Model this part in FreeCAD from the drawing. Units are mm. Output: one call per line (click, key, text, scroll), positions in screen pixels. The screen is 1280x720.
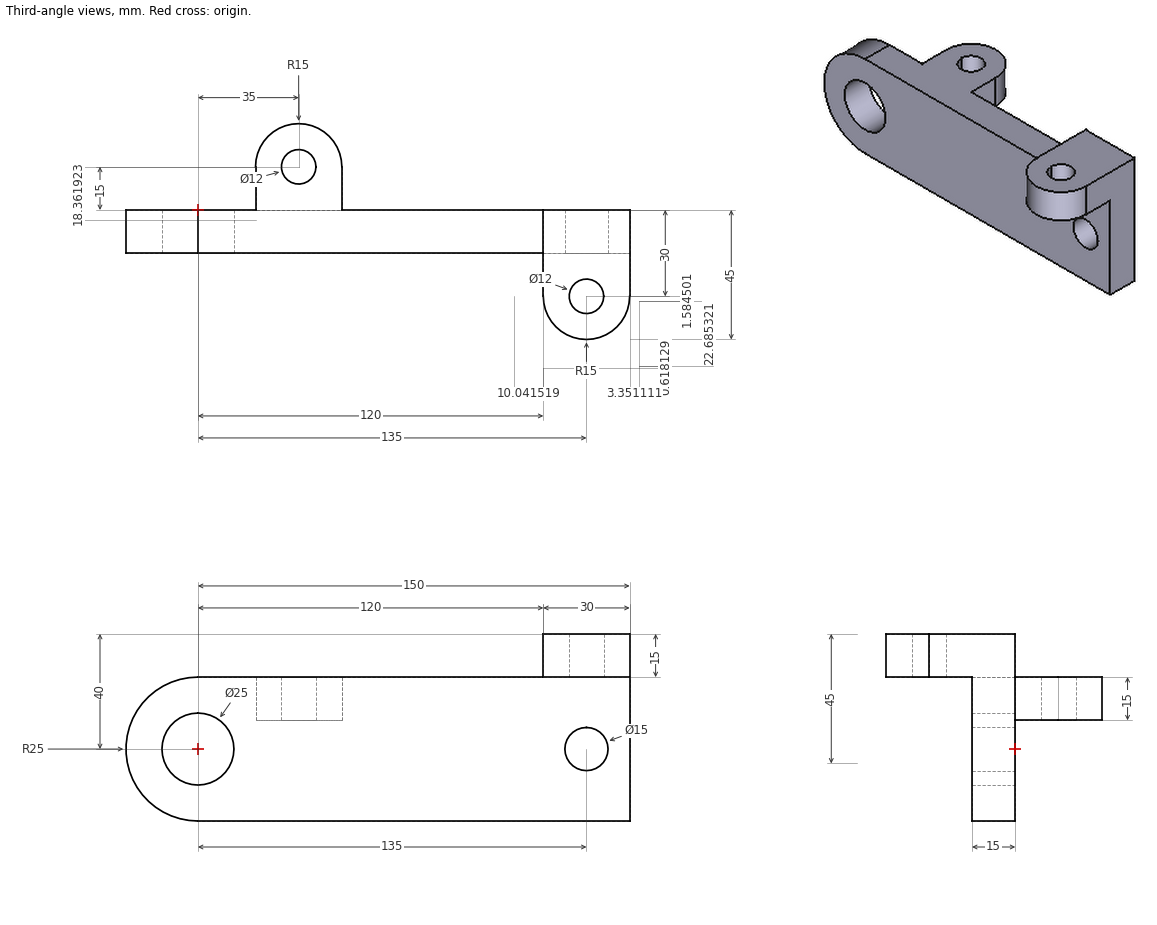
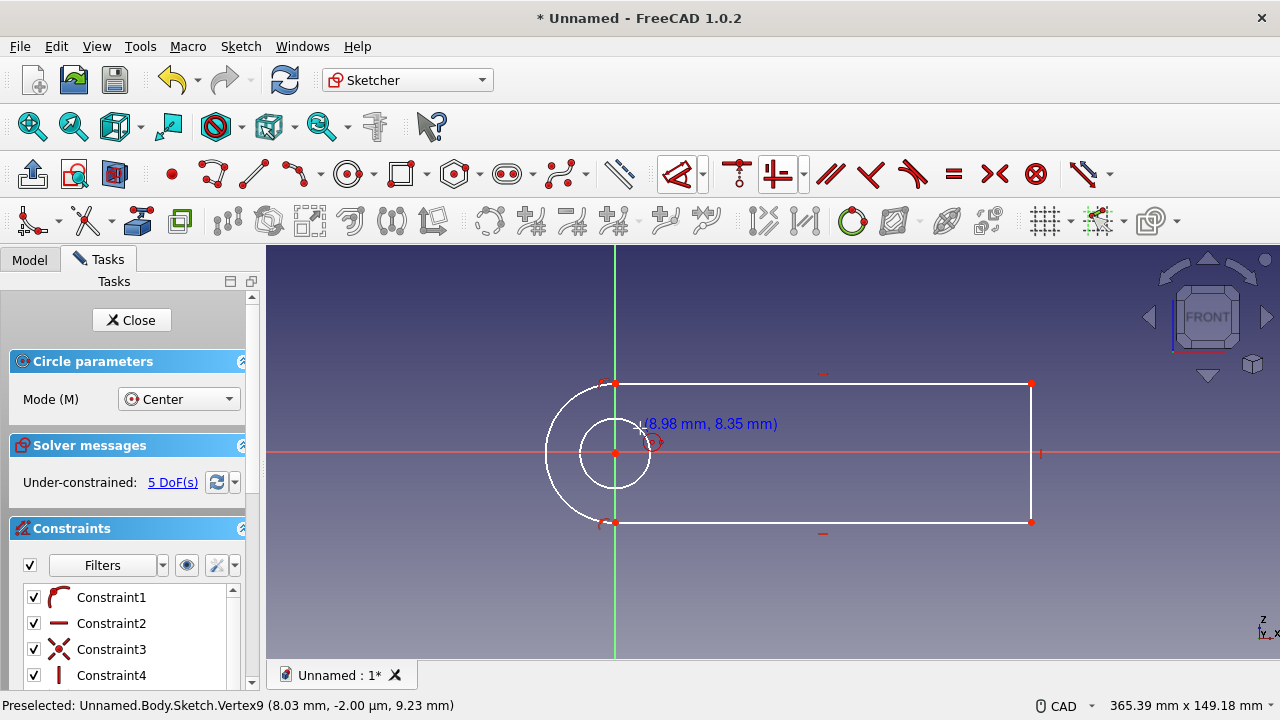
click(990, 452)
click(1004, 437)
key(Escape)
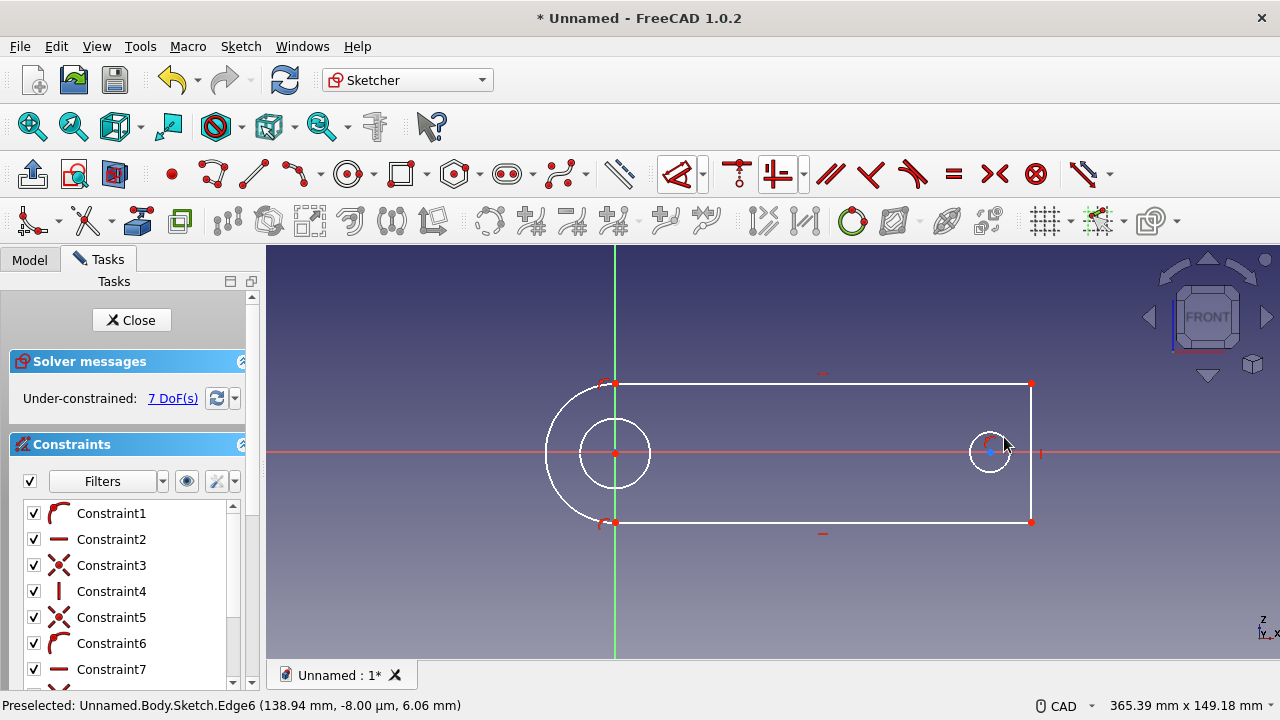
scroll(615, 453, up, 4)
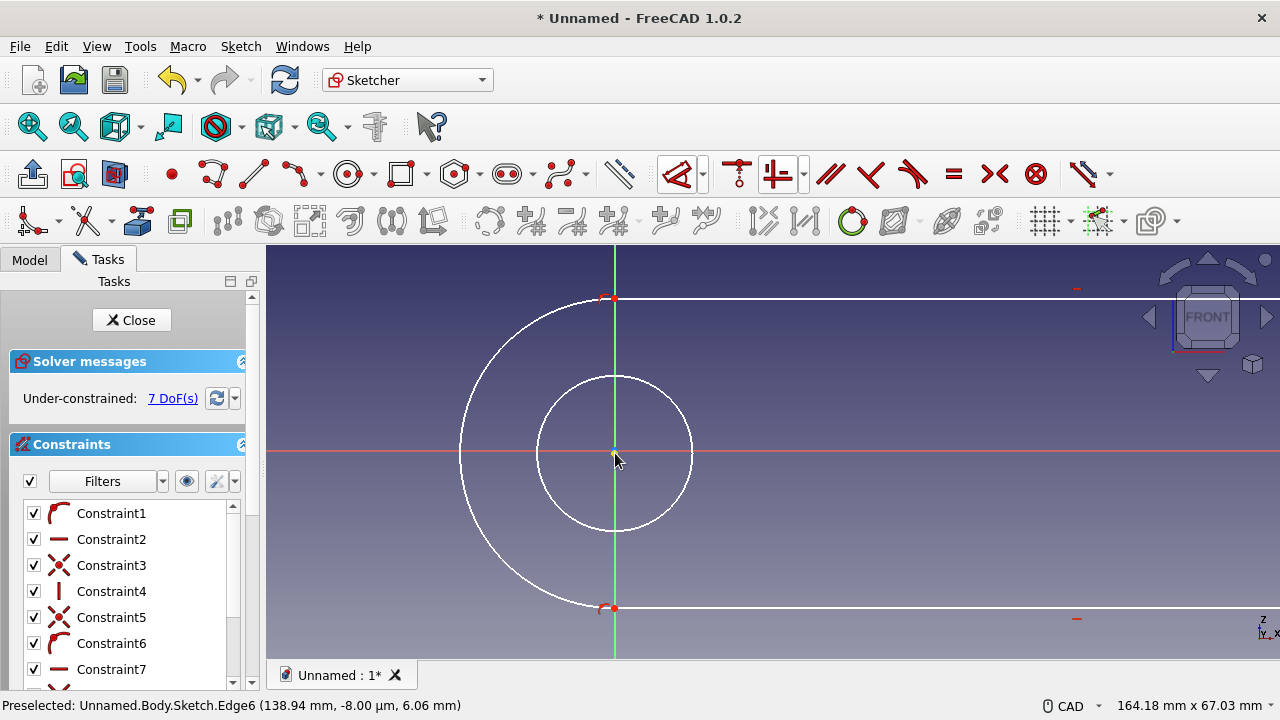
drag(605, 441, 625, 463)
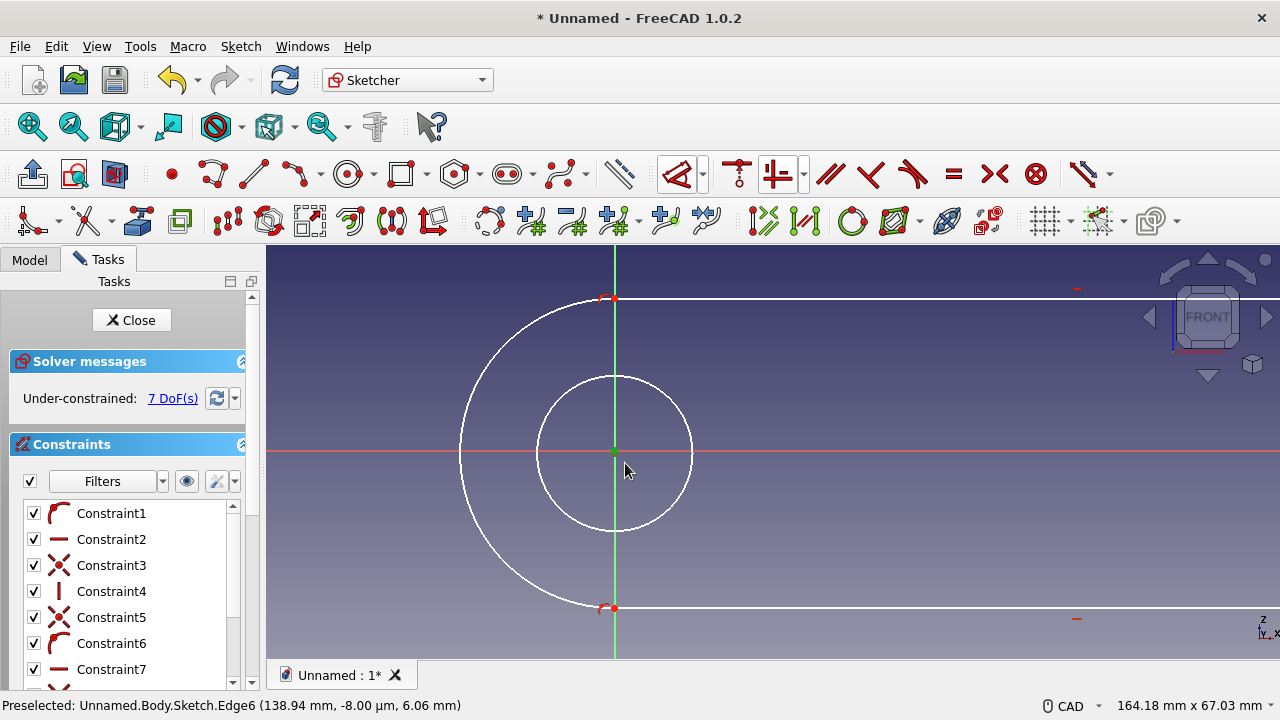
click(737, 174)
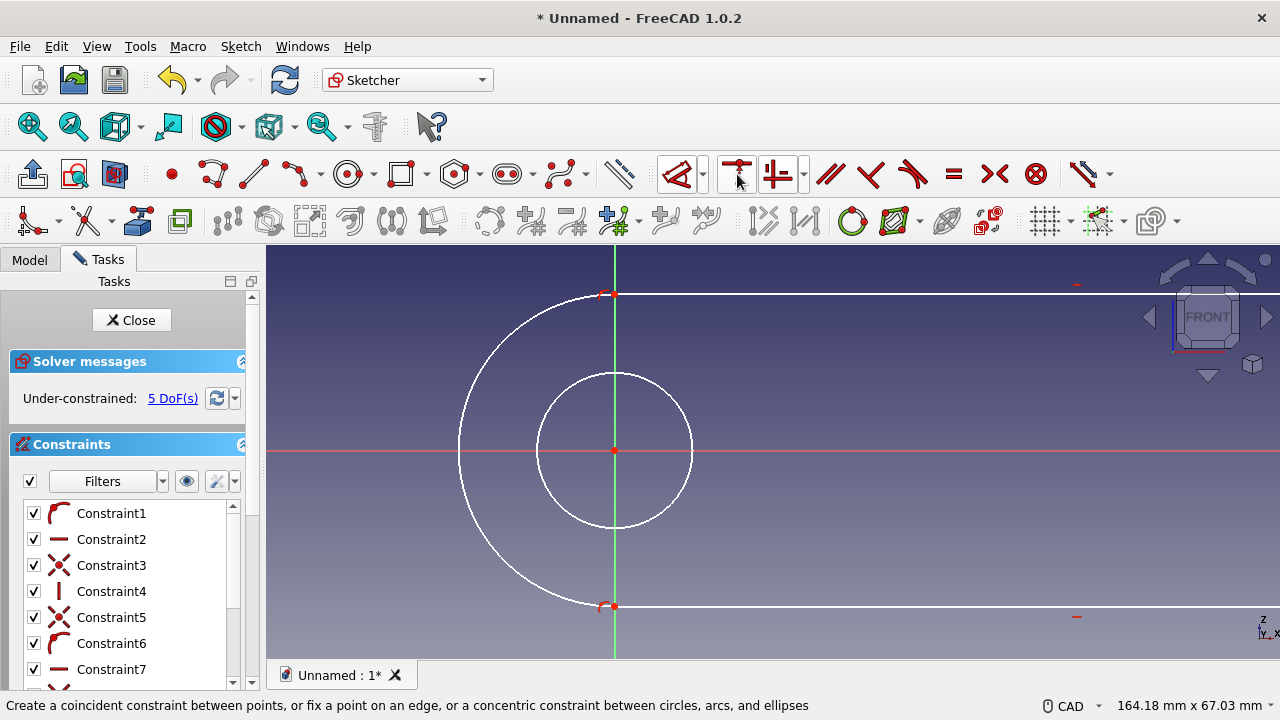
click(488, 359)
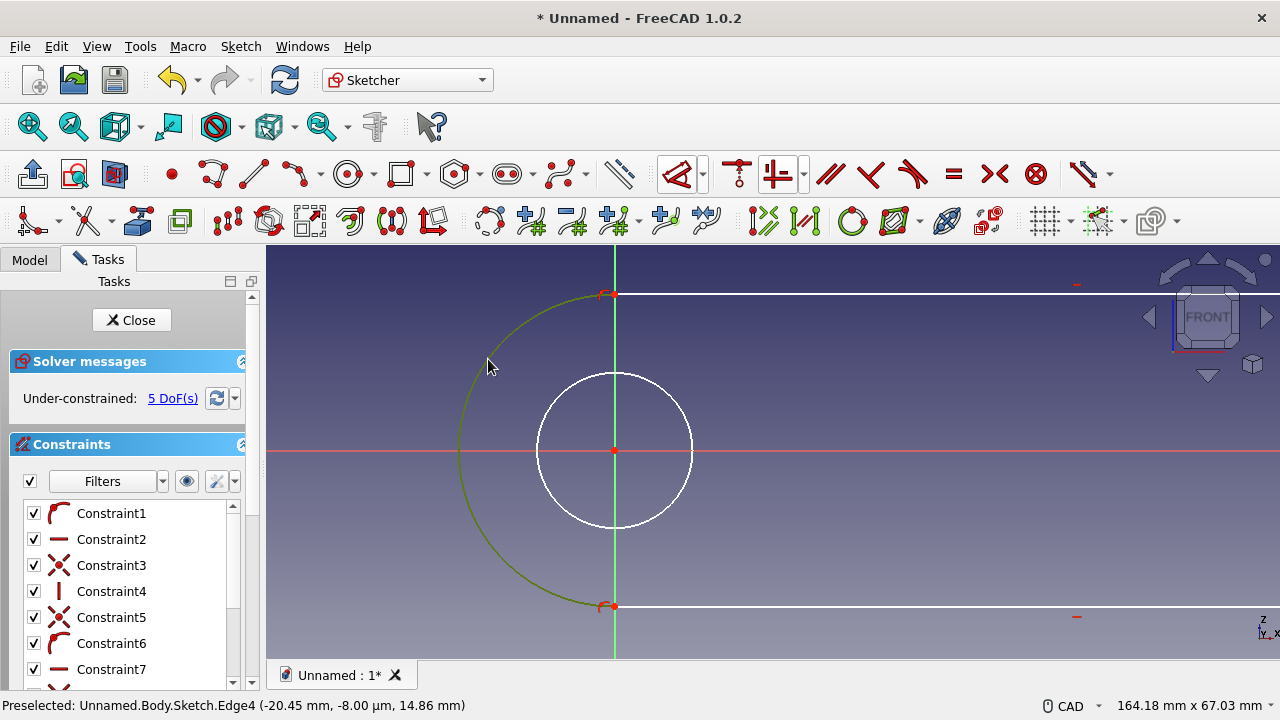
key(k)
key(r)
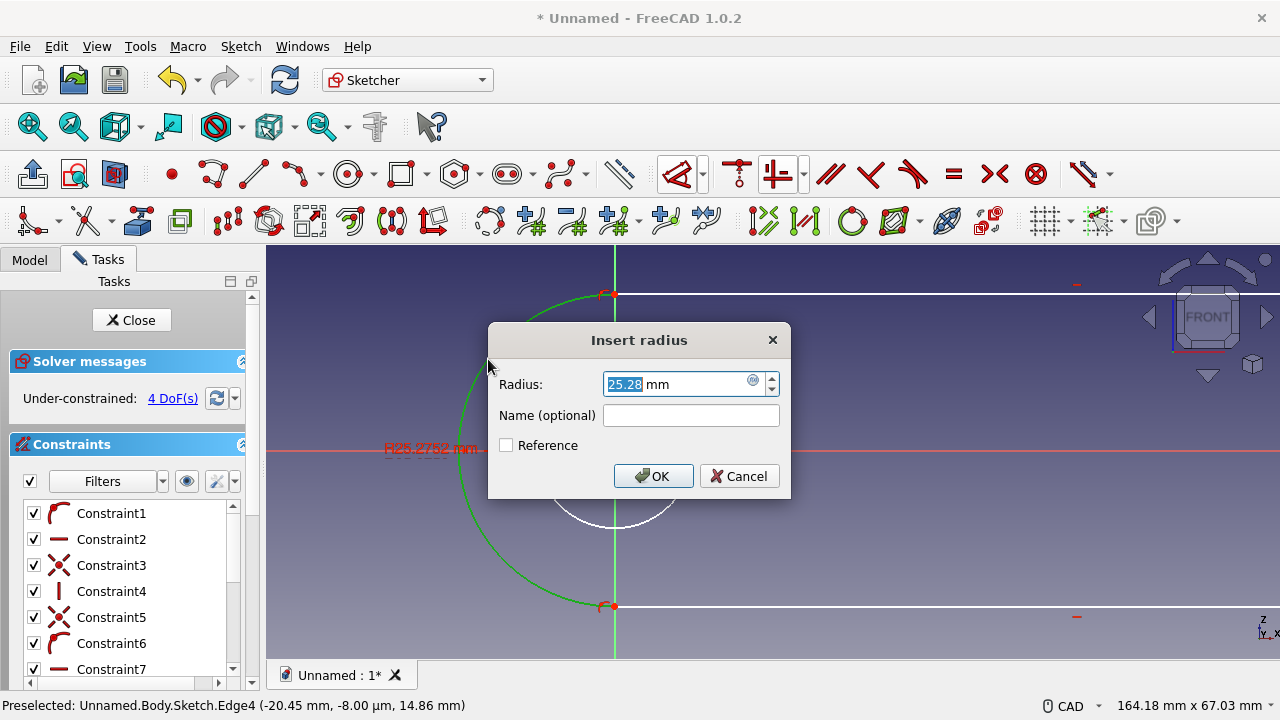
text(25)
key(Return)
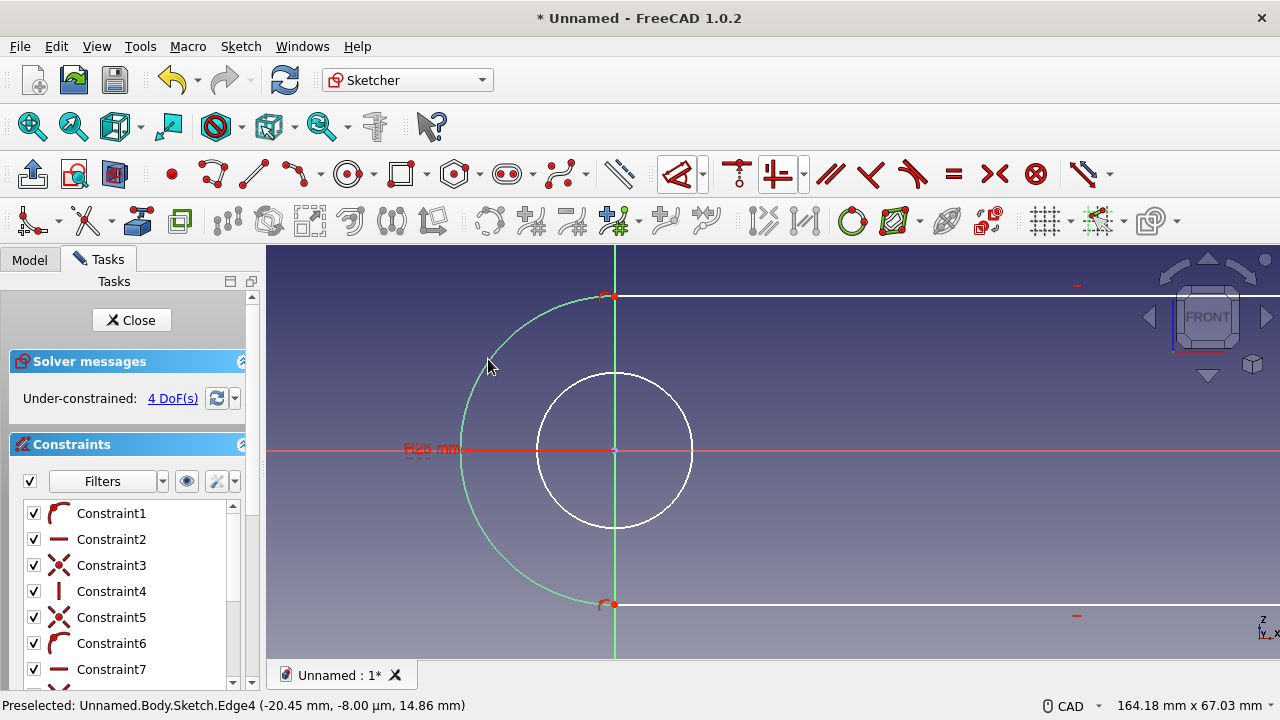
click(670, 395)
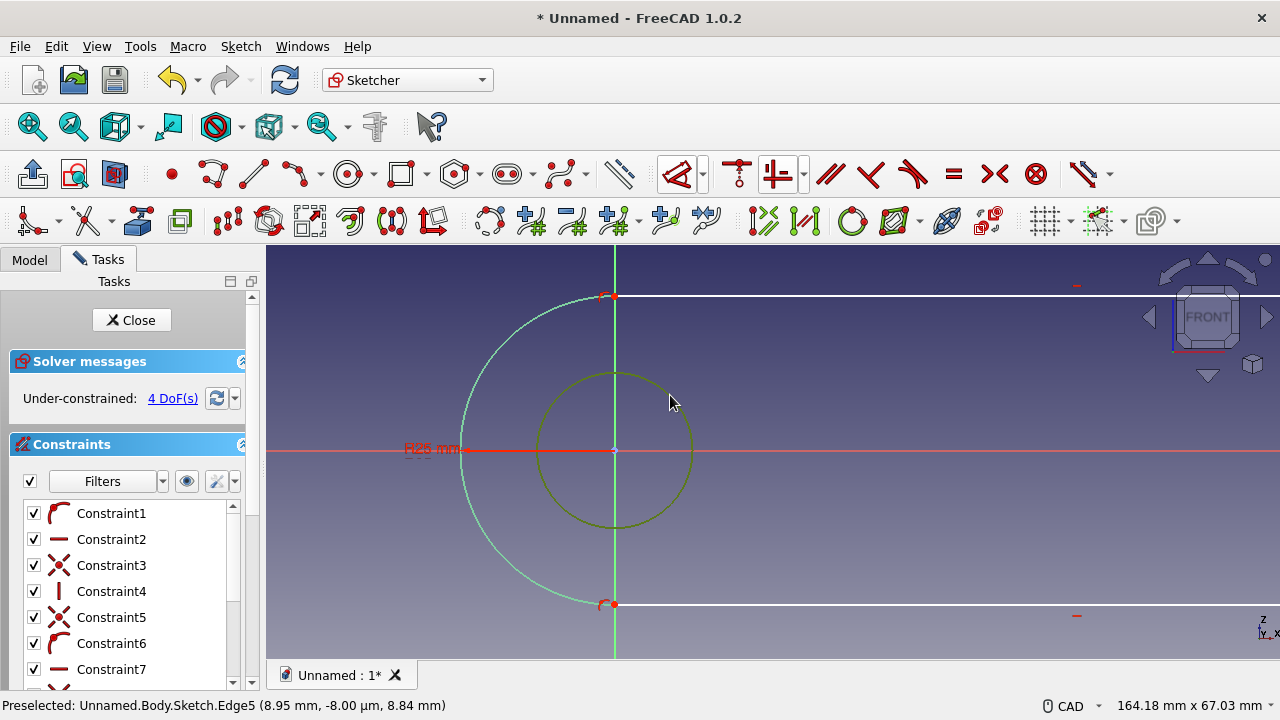
click(702, 174)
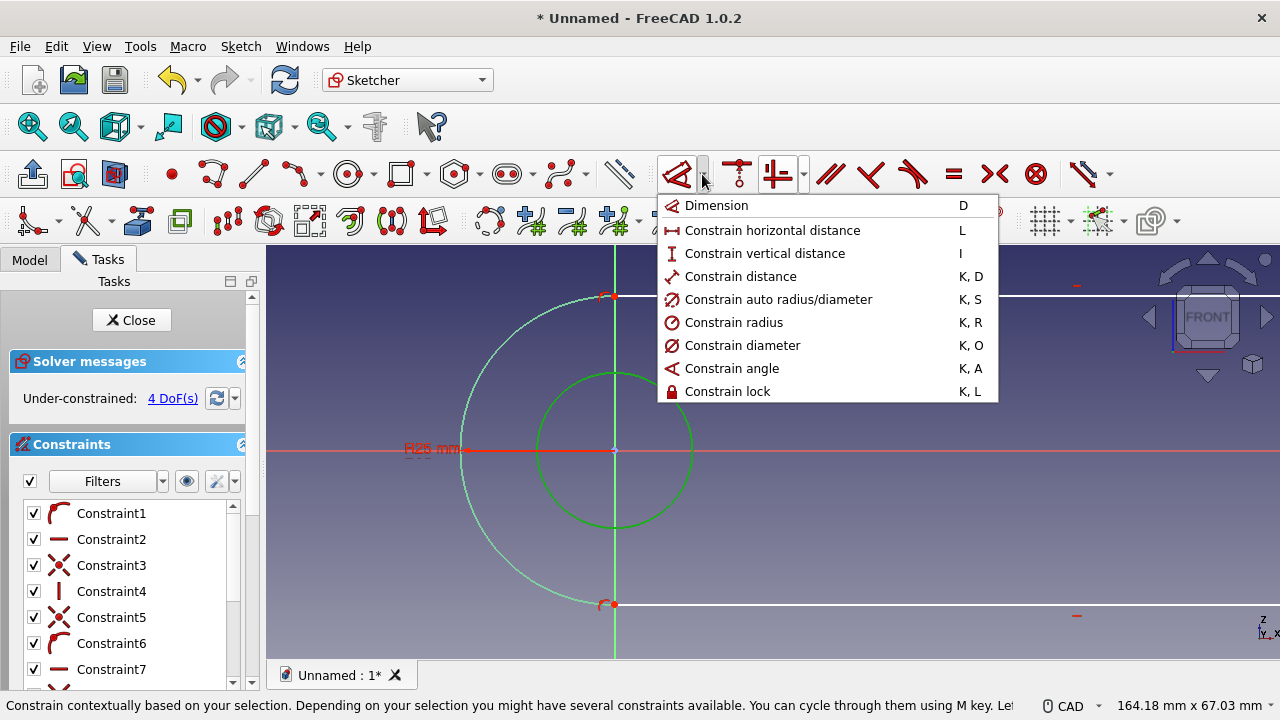
click(828, 346)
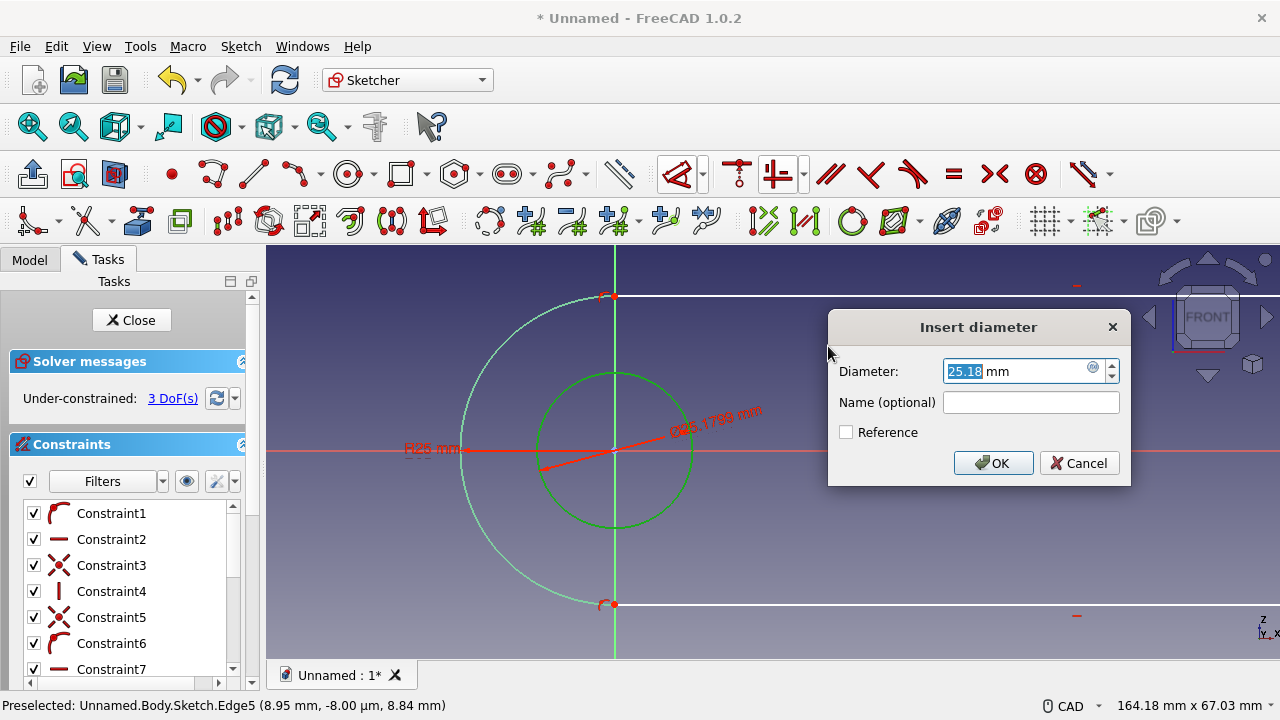
text(25)
key(Return)